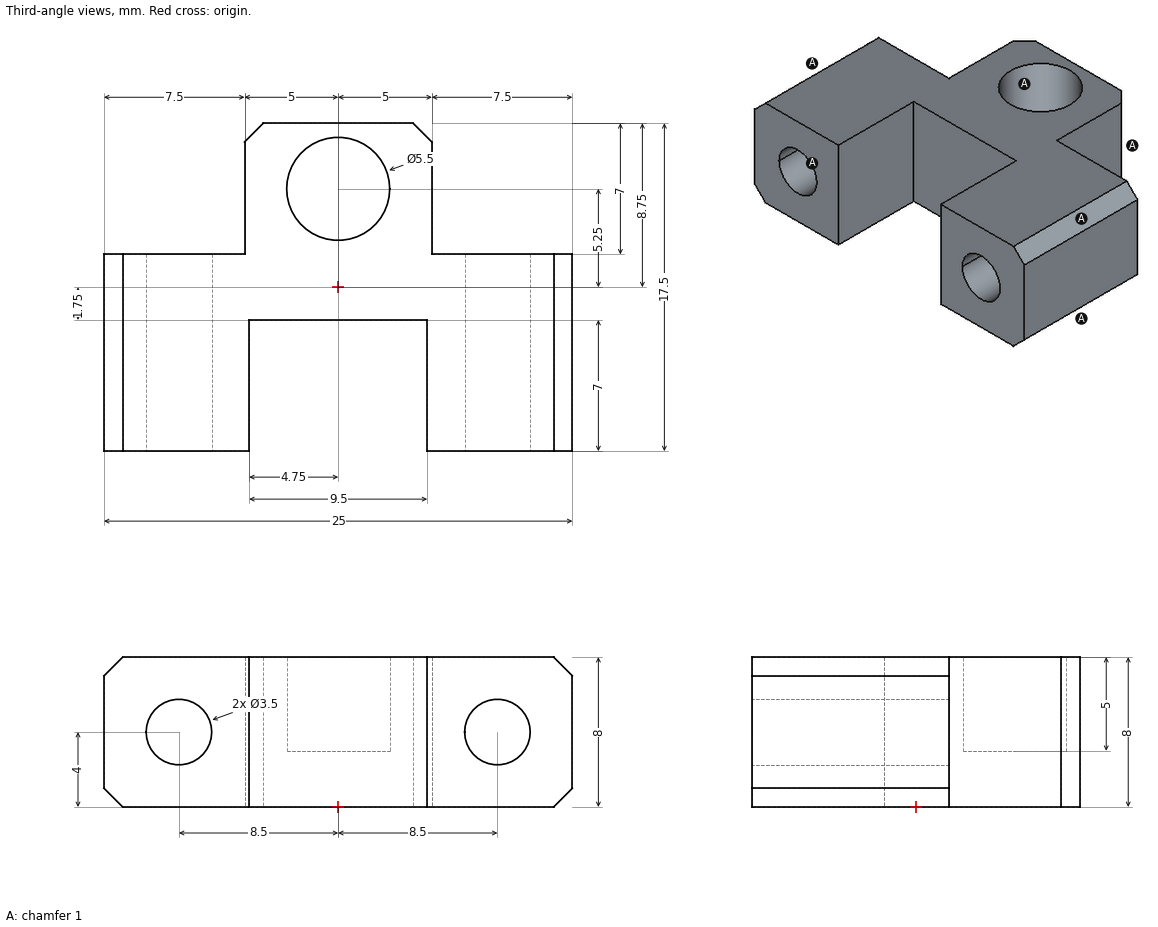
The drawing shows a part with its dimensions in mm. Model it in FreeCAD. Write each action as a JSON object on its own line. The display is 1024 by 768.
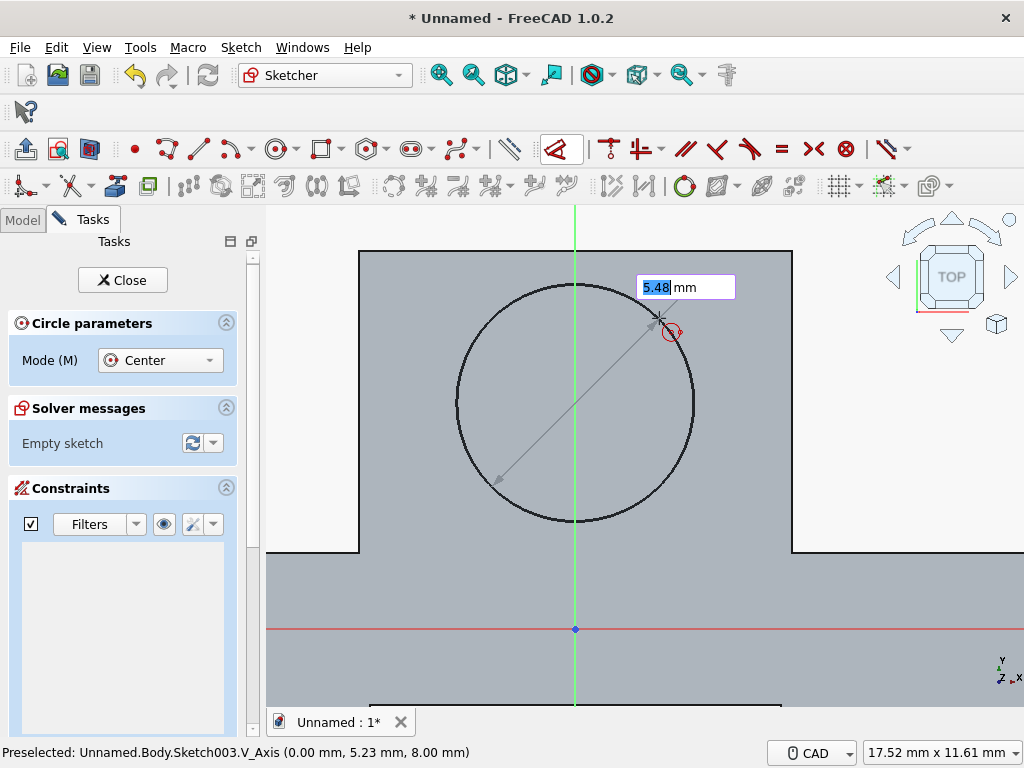
{"action": "type", "text": "5.5"}
{"action": "key", "text": "Return"}
{"action": "key", "text": "Escape"}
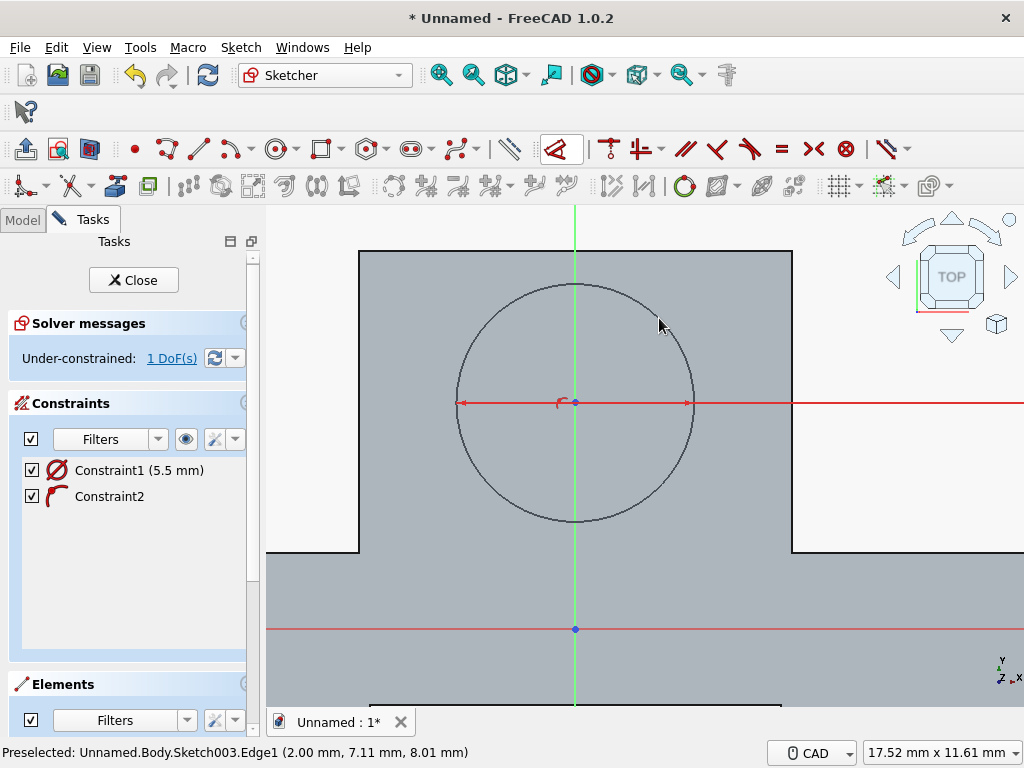
{"action": "left_click", "coordinate": [575, 403]}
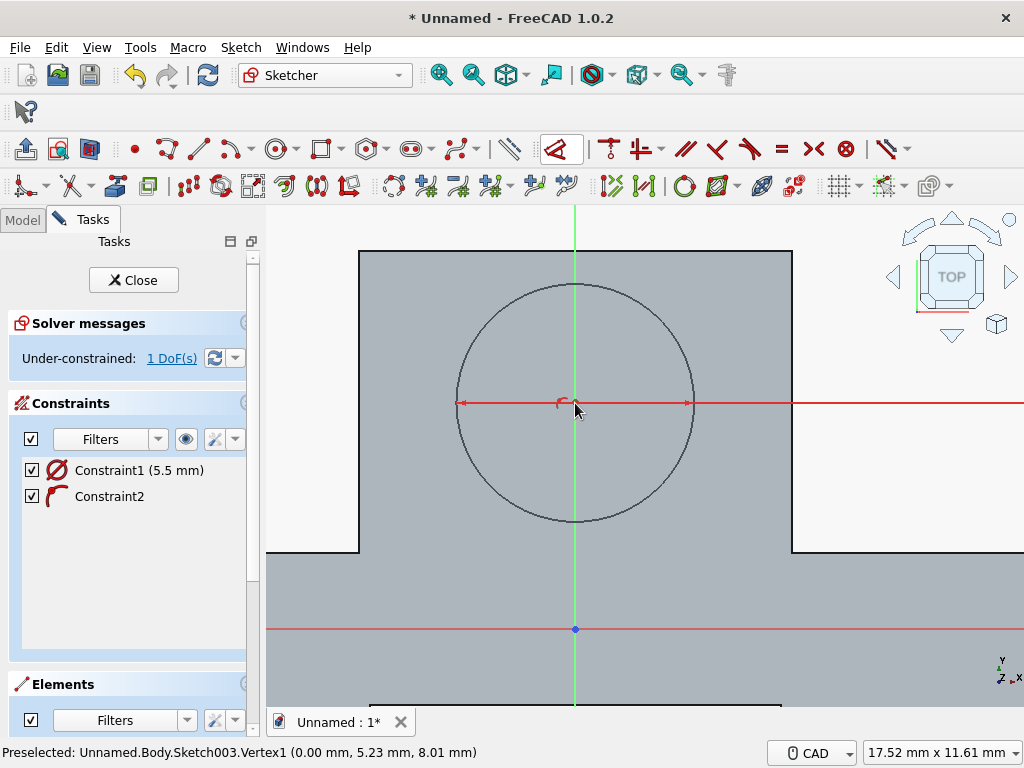
{"action": "key", "text": "i"}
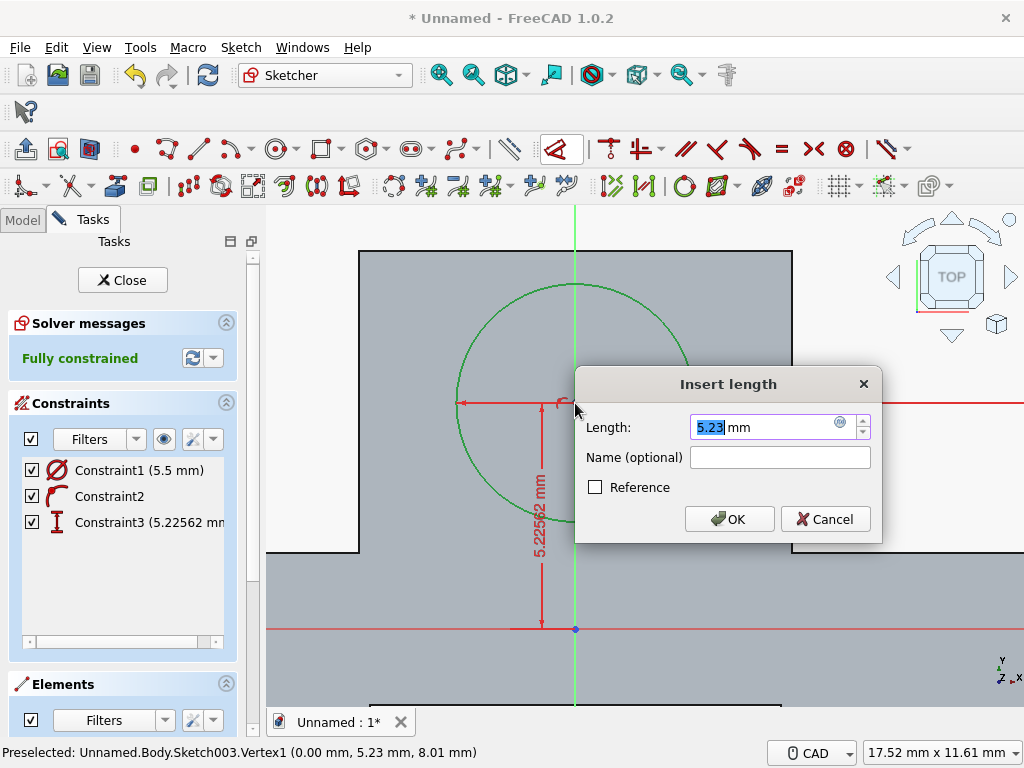
{"action": "type", "text": "5.25"}
{"action": "key", "text": "Return"}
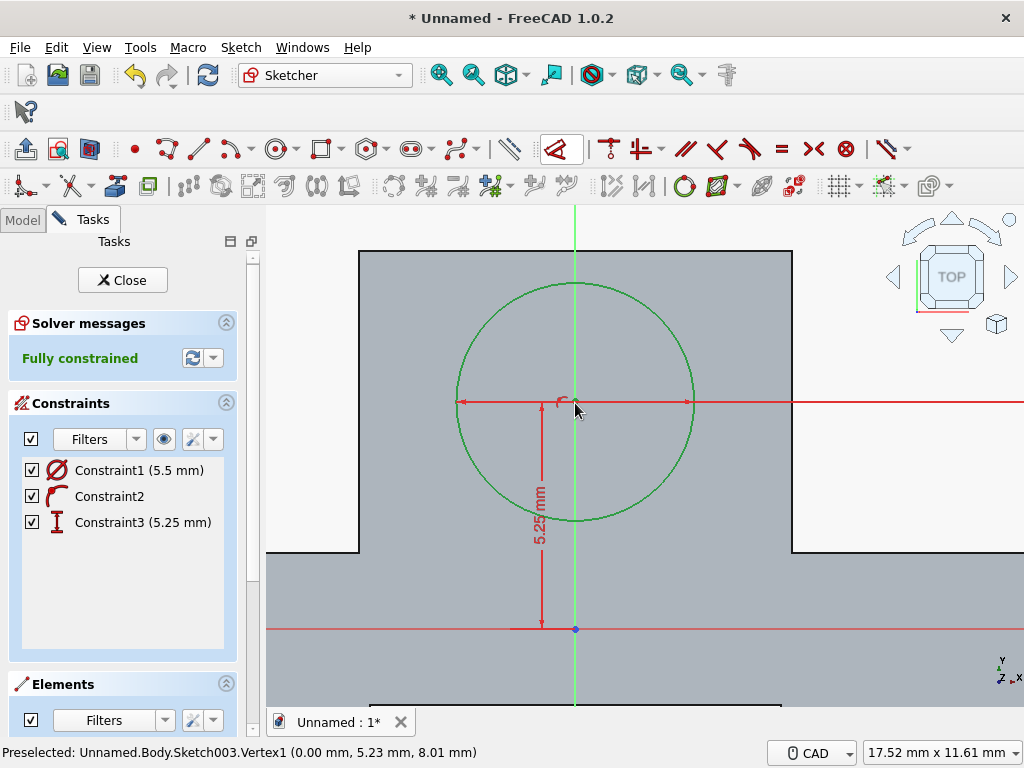
{"action": "left_click", "coordinate": [123, 280]}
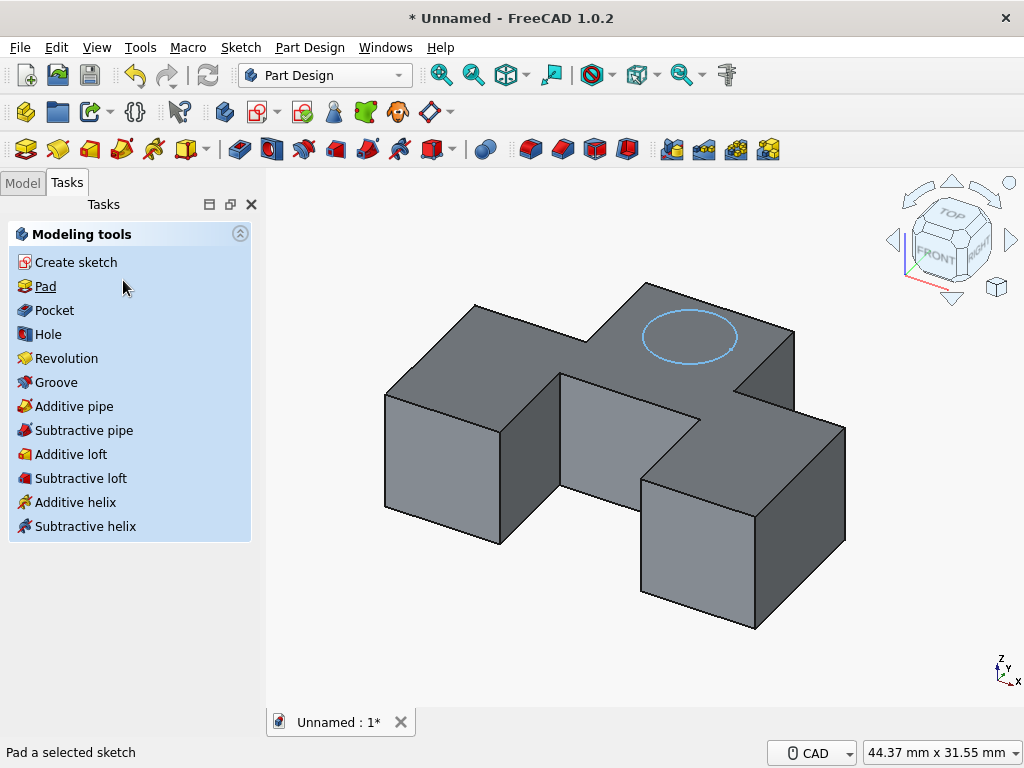
{"action": "left_click", "coordinate": [240, 150]}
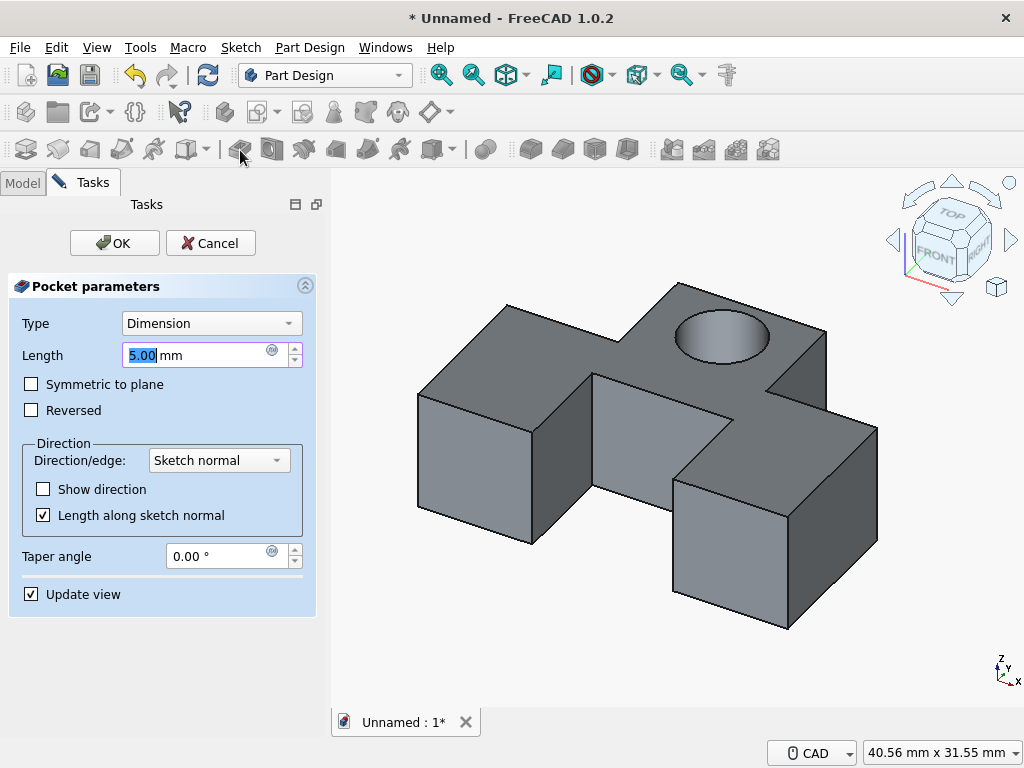
{"action": "type", "text": "5"}
{"action": "key", "text": "Tab"}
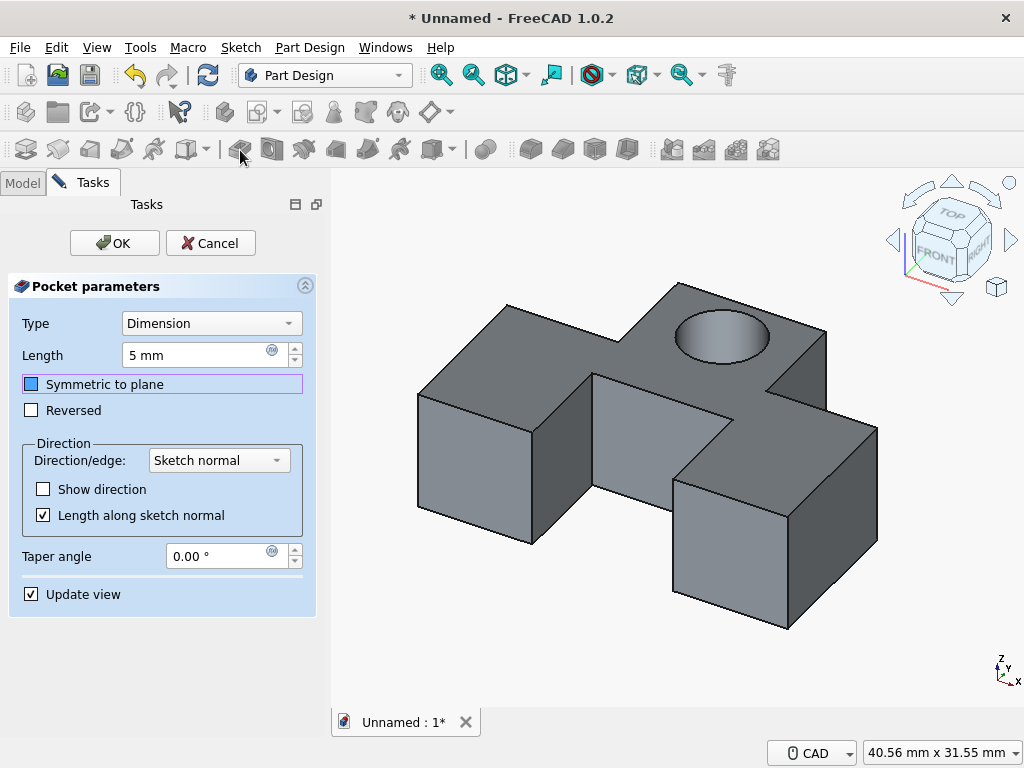
{"action": "left_click", "coordinate": [115, 243]}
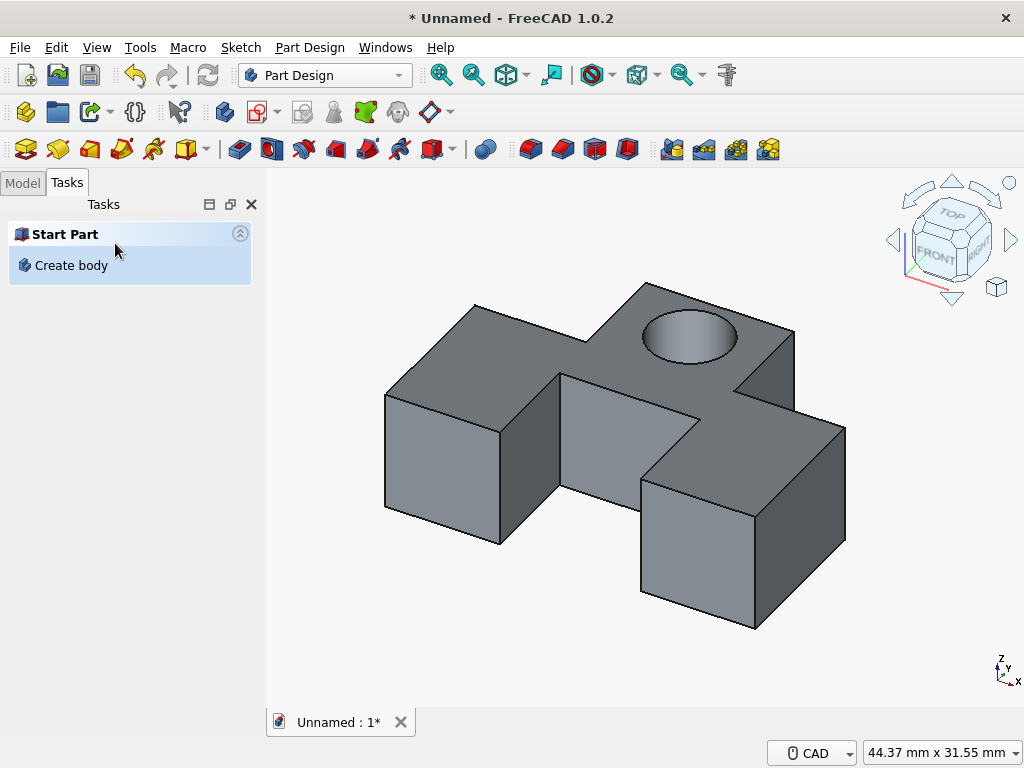
{"action": "key", "text": "4"}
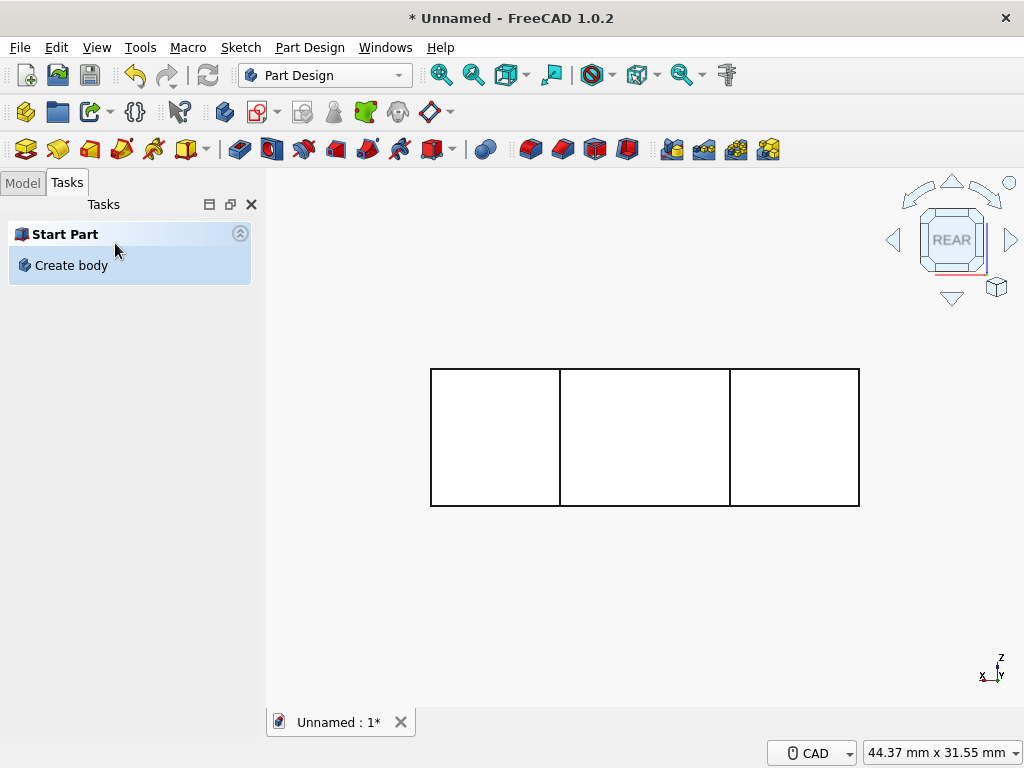
{"action": "left_click", "coordinate": [794, 436]}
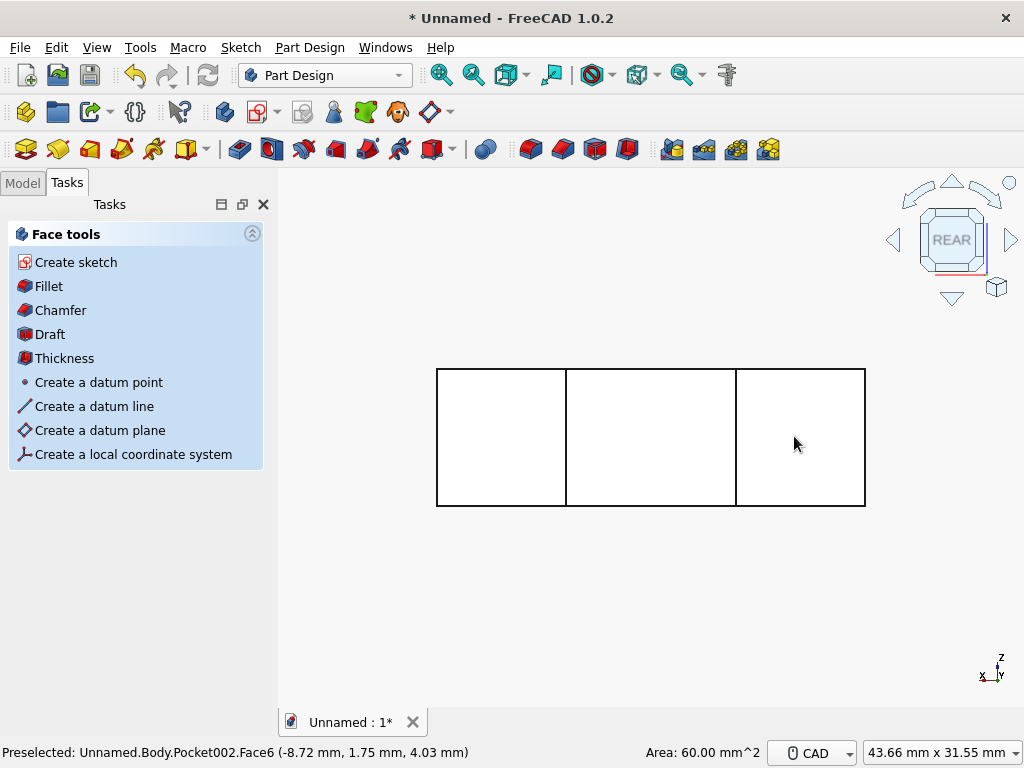
{"action": "left_click", "coordinate": [258, 112]}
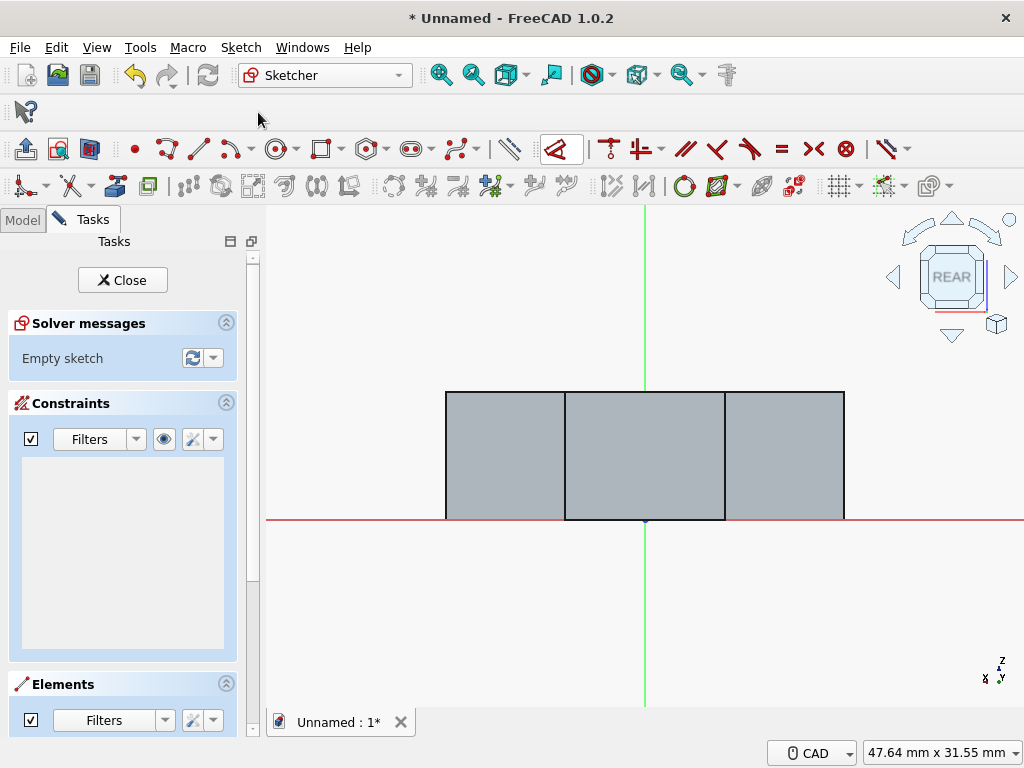
{"action": "left_click", "coordinate": [90, 150]}